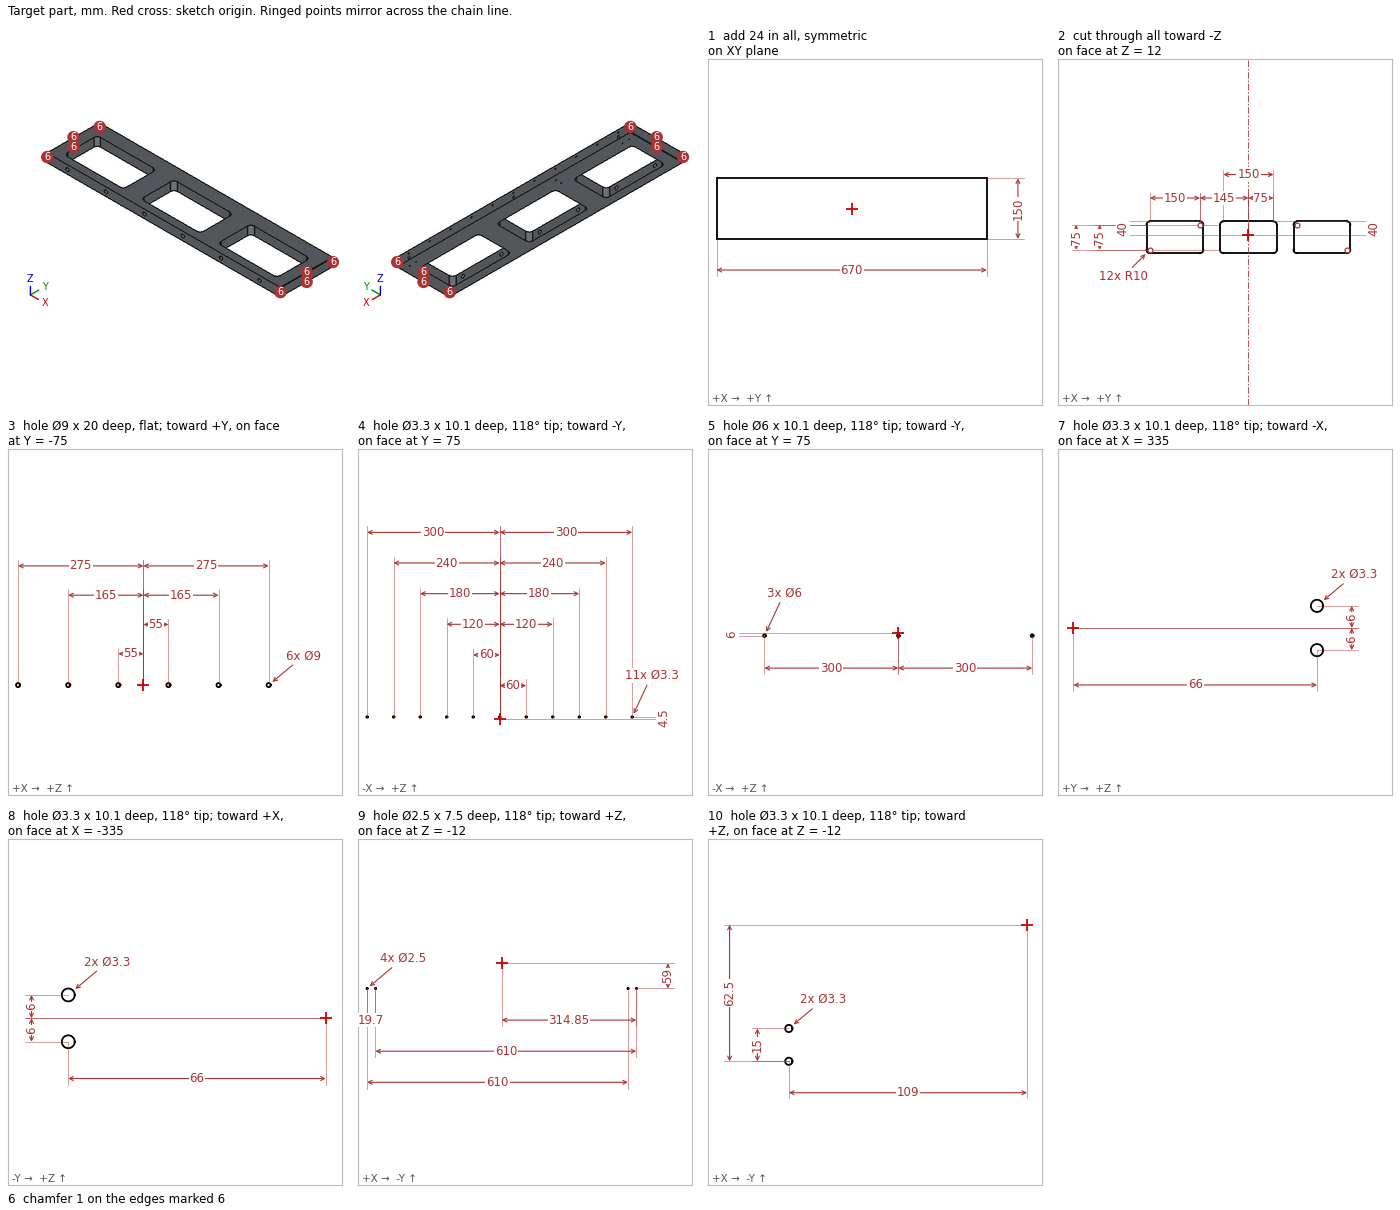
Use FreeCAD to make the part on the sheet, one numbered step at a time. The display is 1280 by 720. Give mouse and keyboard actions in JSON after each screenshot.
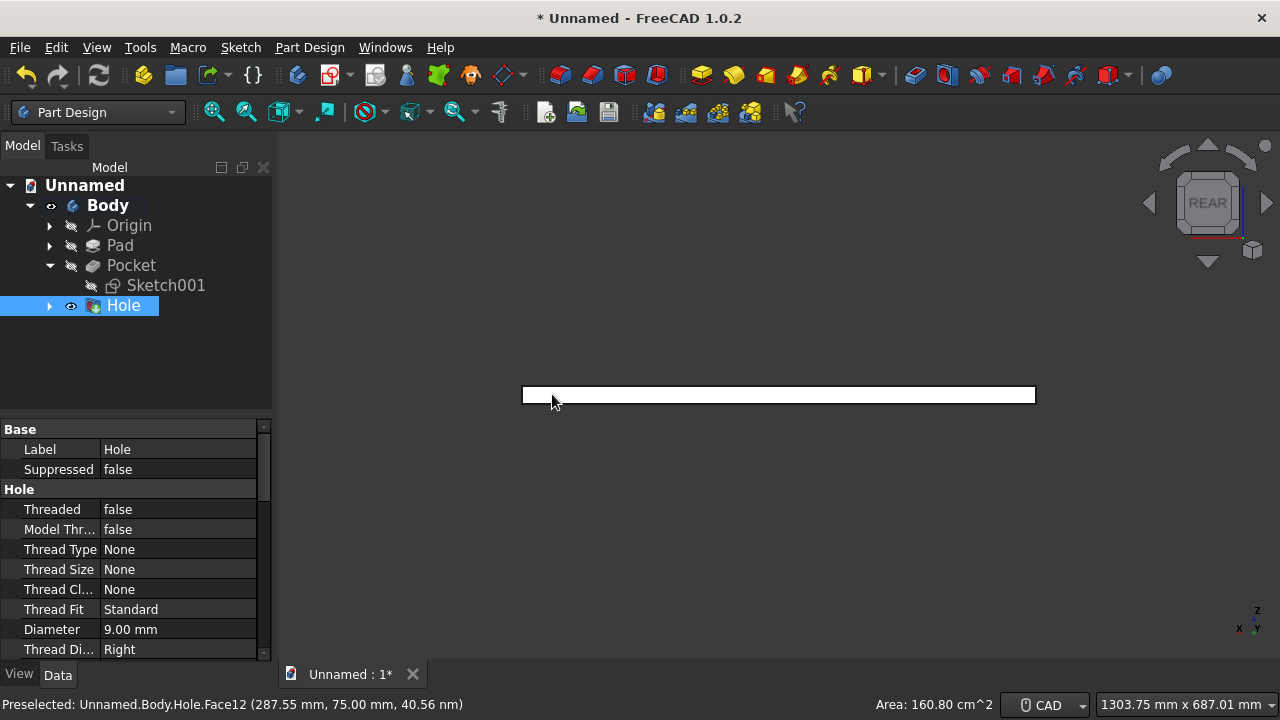
{"action": "left_click", "coordinate": [330, 76]}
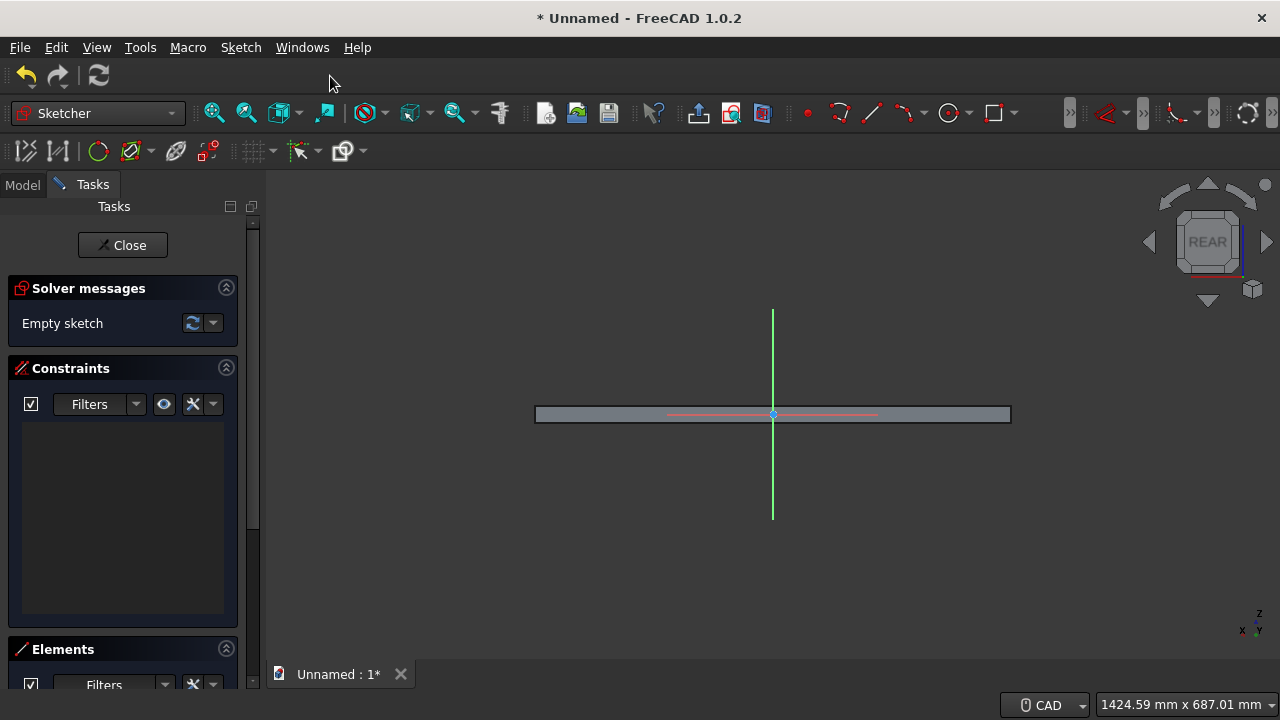
{"action": "left_click", "coordinate": [950, 114]}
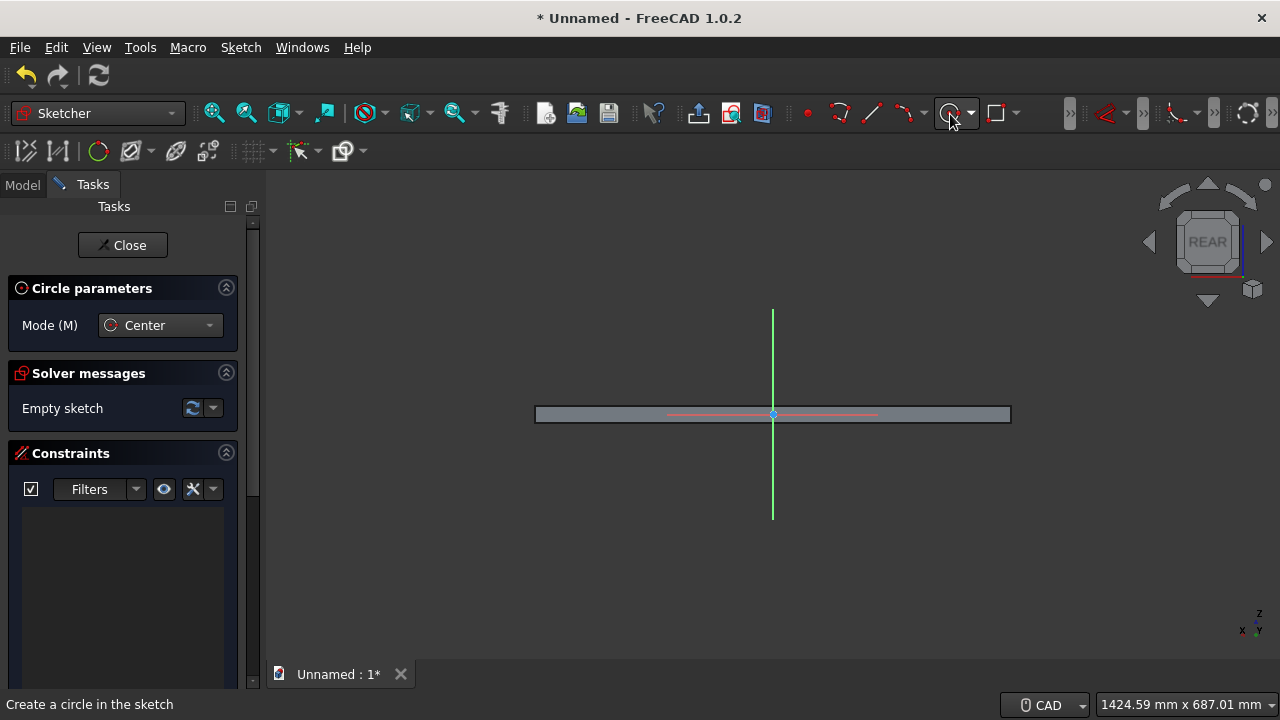
{"action": "scroll", "coordinate": [987, 411], "scroll_direction": "up", "scroll_amount": 15}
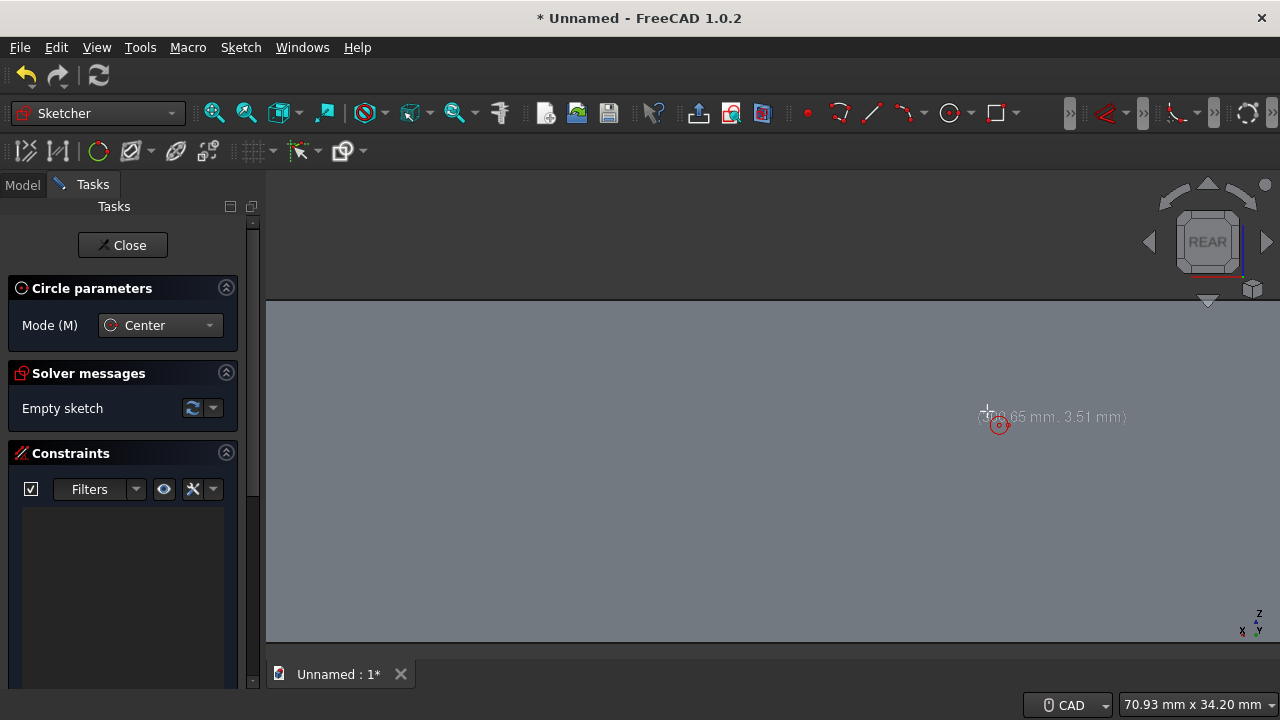
{"action": "scroll", "coordinate": [965, 414], "scroll_direction": "down", "scroll_amount": 14}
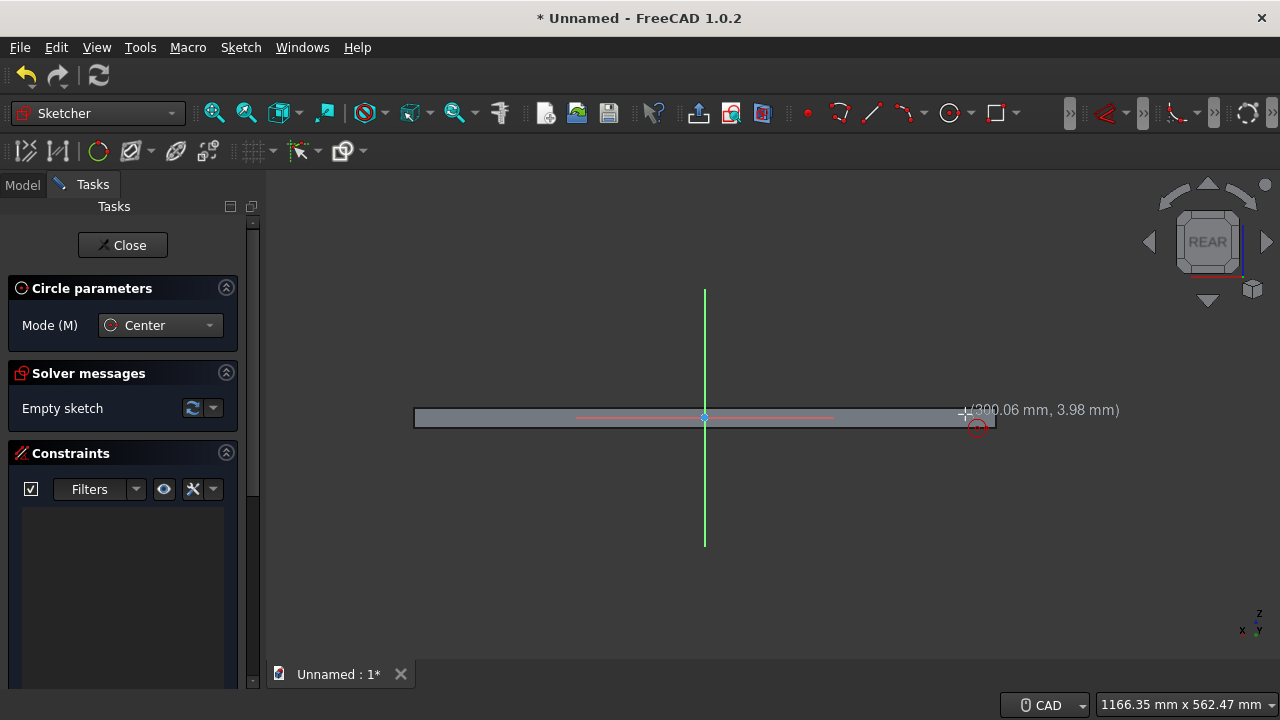
{"action": "scroll", "coordinate": [966, 414], "scroll_direction": "up", "scroll_amount": 8}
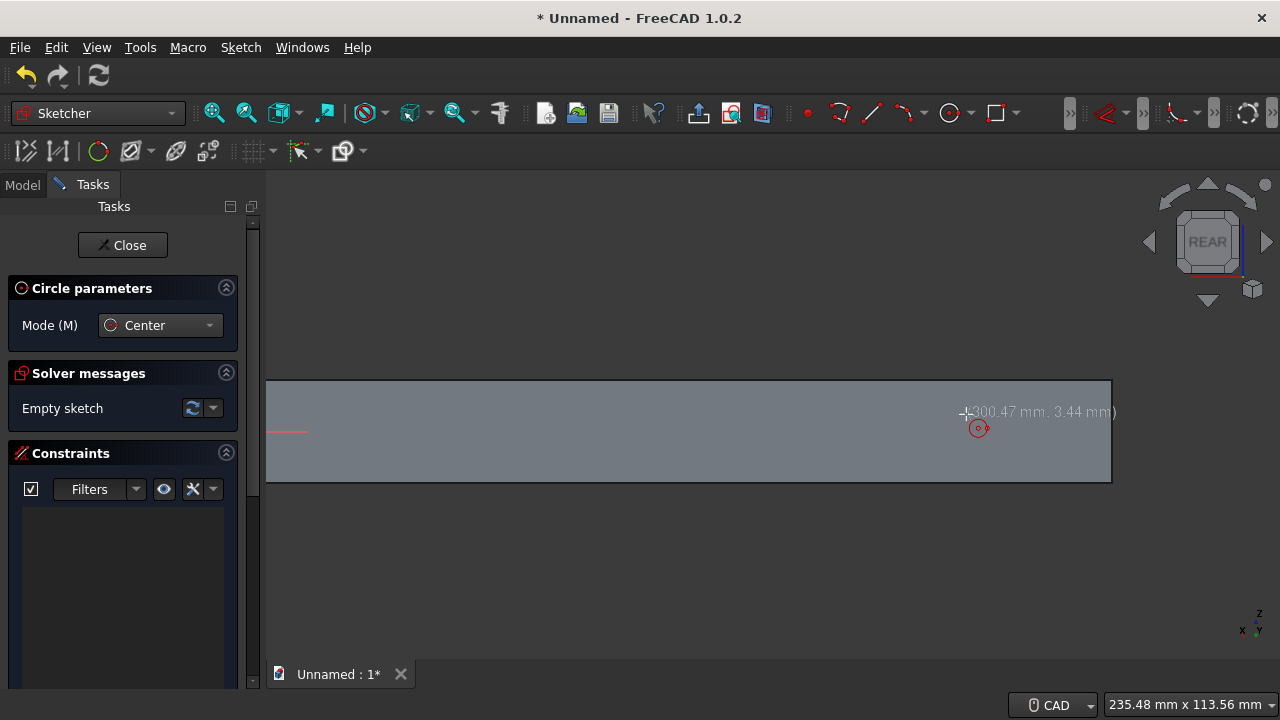
{"action": "left_click", "coordinate": [961, 412]}
{"action": "mouse_move", "coordinate": [966, 407]}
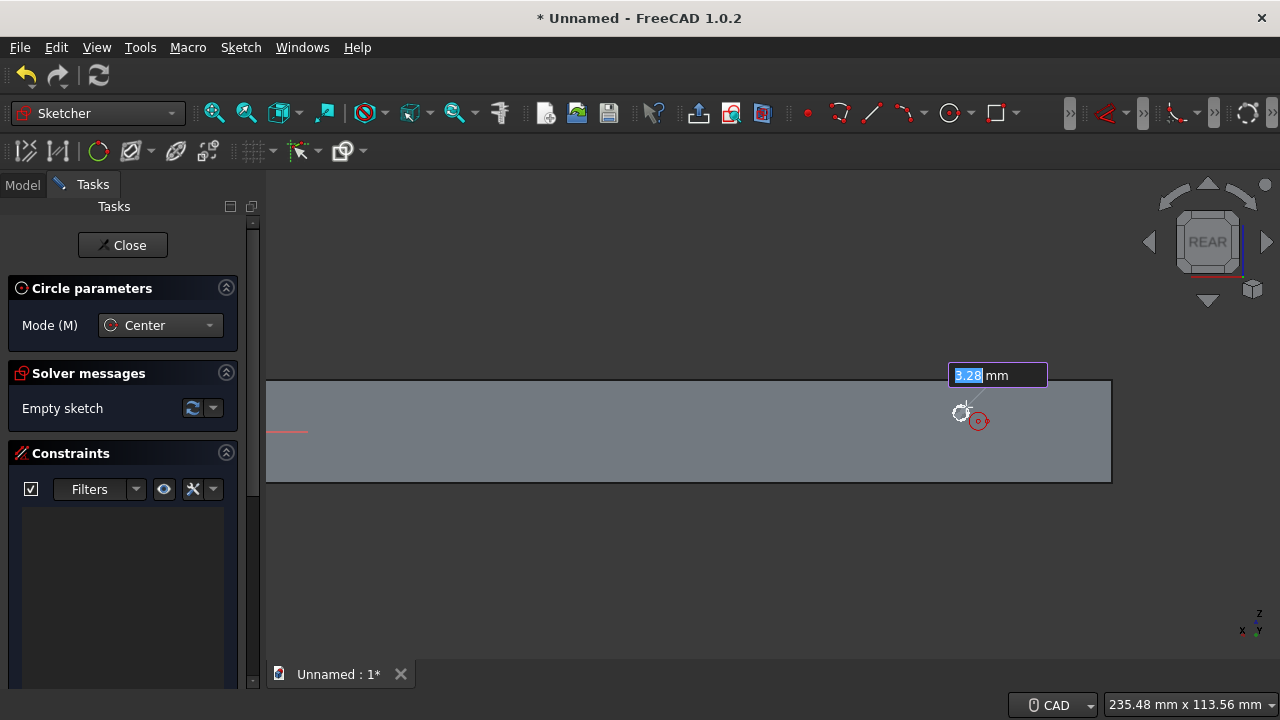
{"action": "type", "text": "3.3"}
{"action": "key", "text": "Return"}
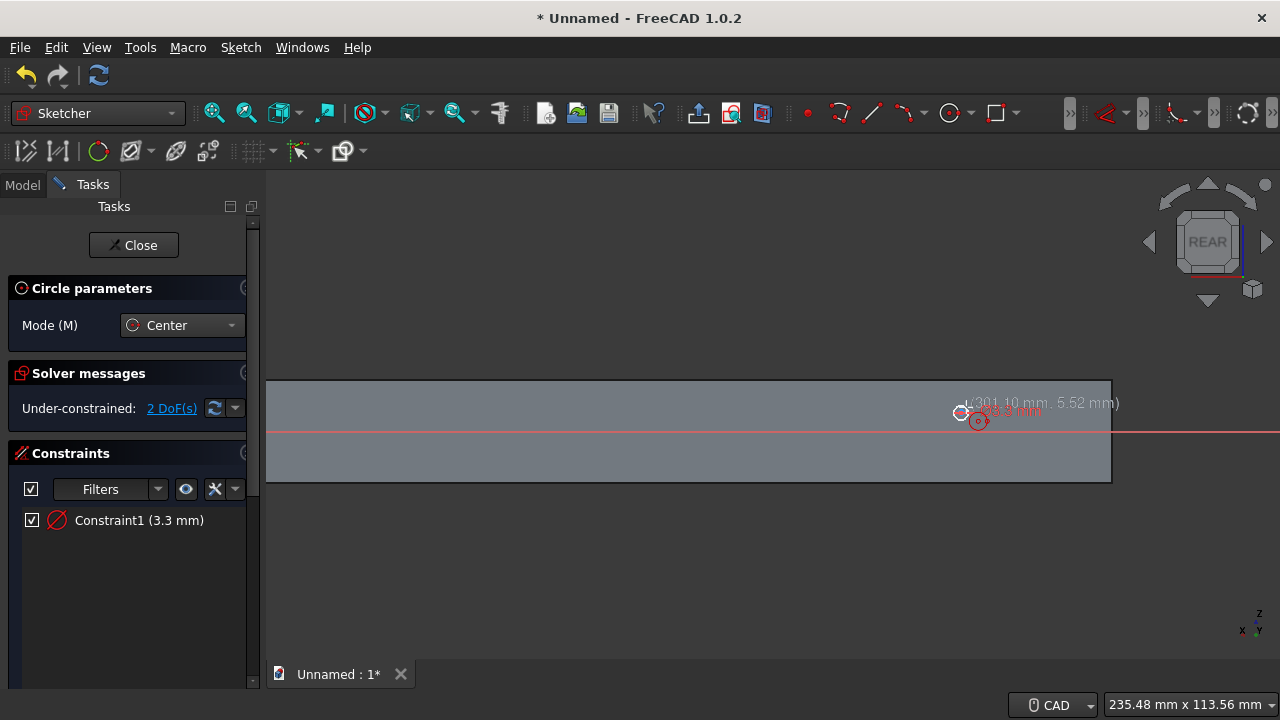
{"action": "scroll", "coordinate": [703, 412], "scroll_direction": "up", "scroll_amount": 6}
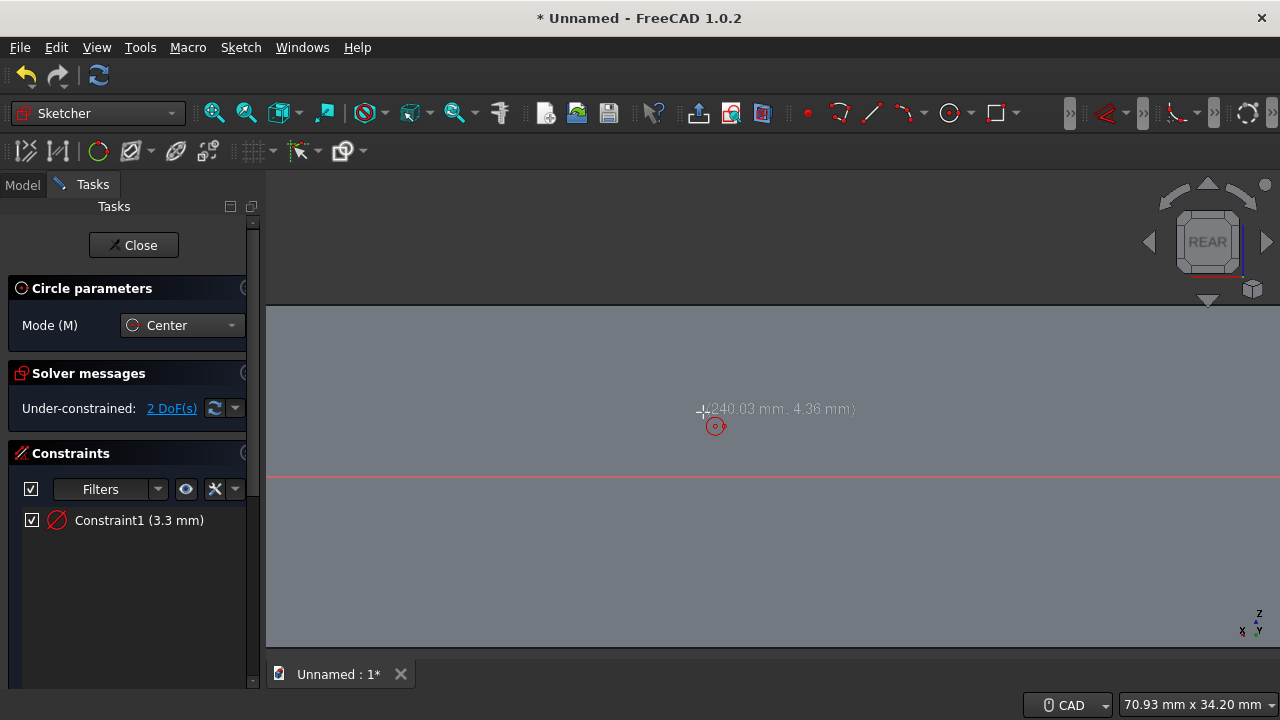
{"action": "scroll", "coordinate": [927, 413], "scroll_direction": "down", "scroll_amount": 14}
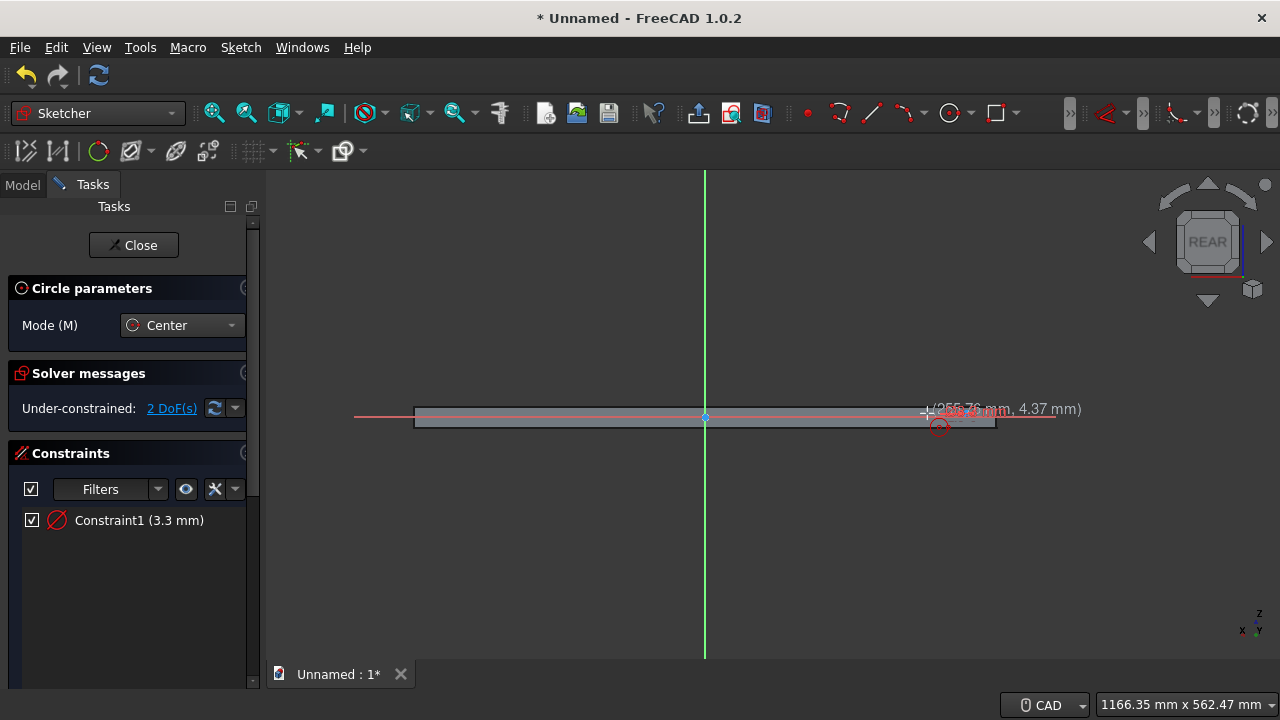
{"action": "scroll", "coordinate": [914, 413], "scroll_direction": "up", "scroll_amount": 8}